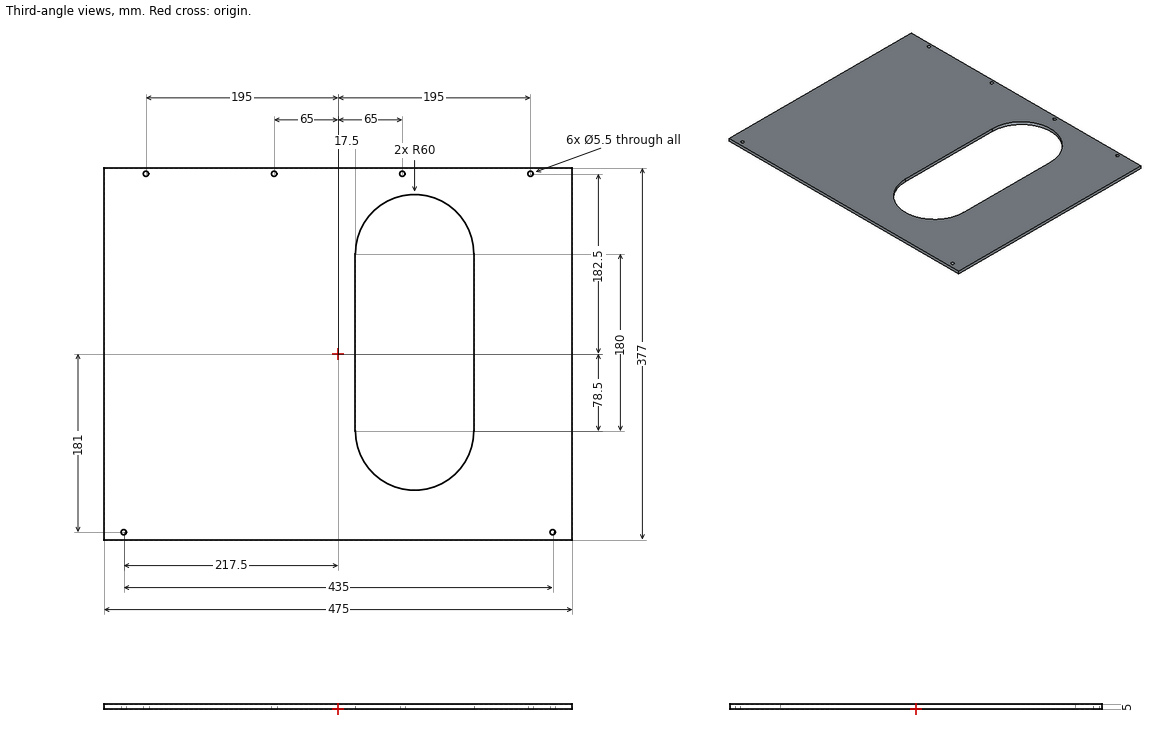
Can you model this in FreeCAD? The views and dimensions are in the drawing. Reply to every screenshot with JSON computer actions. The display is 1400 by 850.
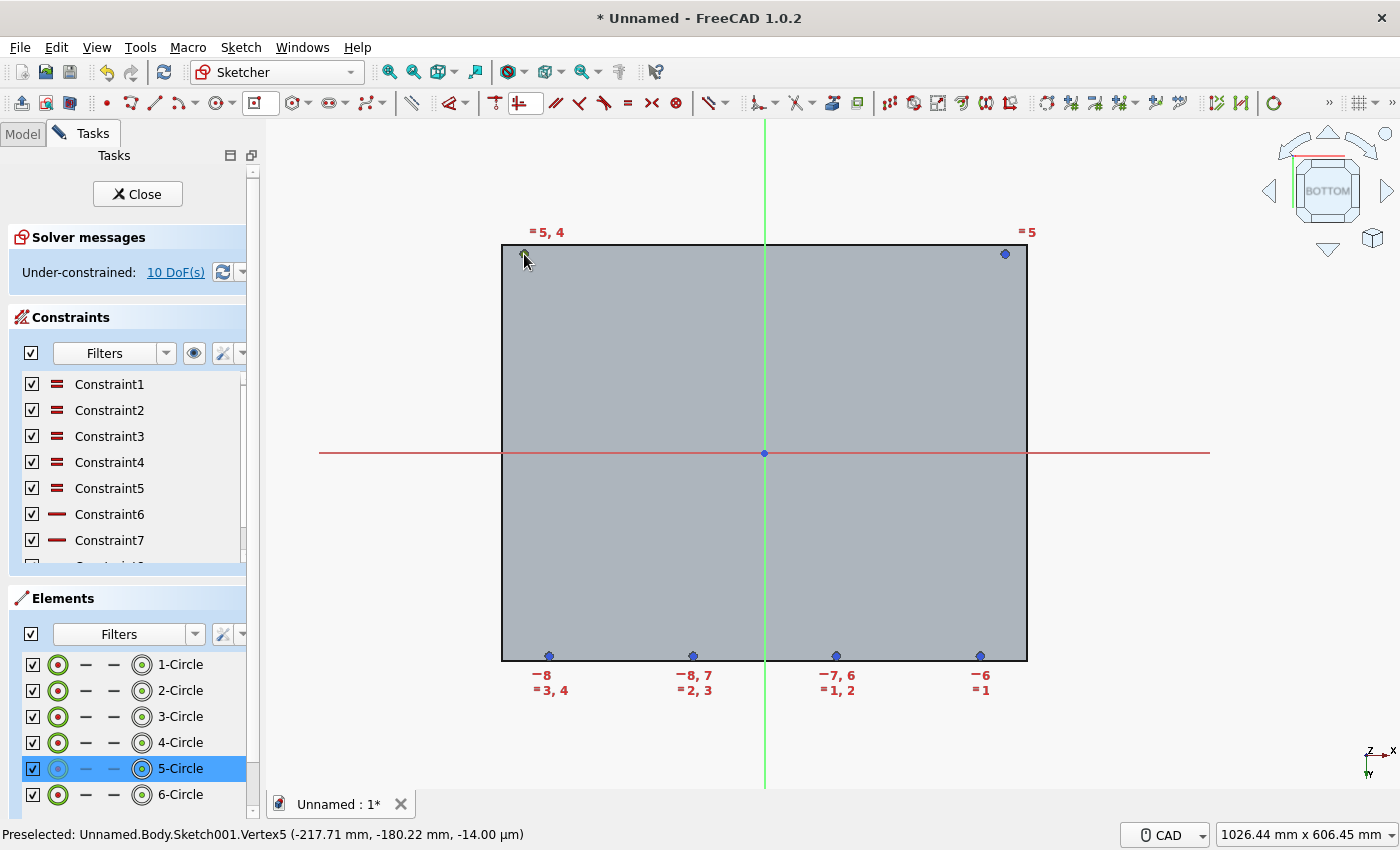
{"action": "left_click", "coordinate": [1005, 254]}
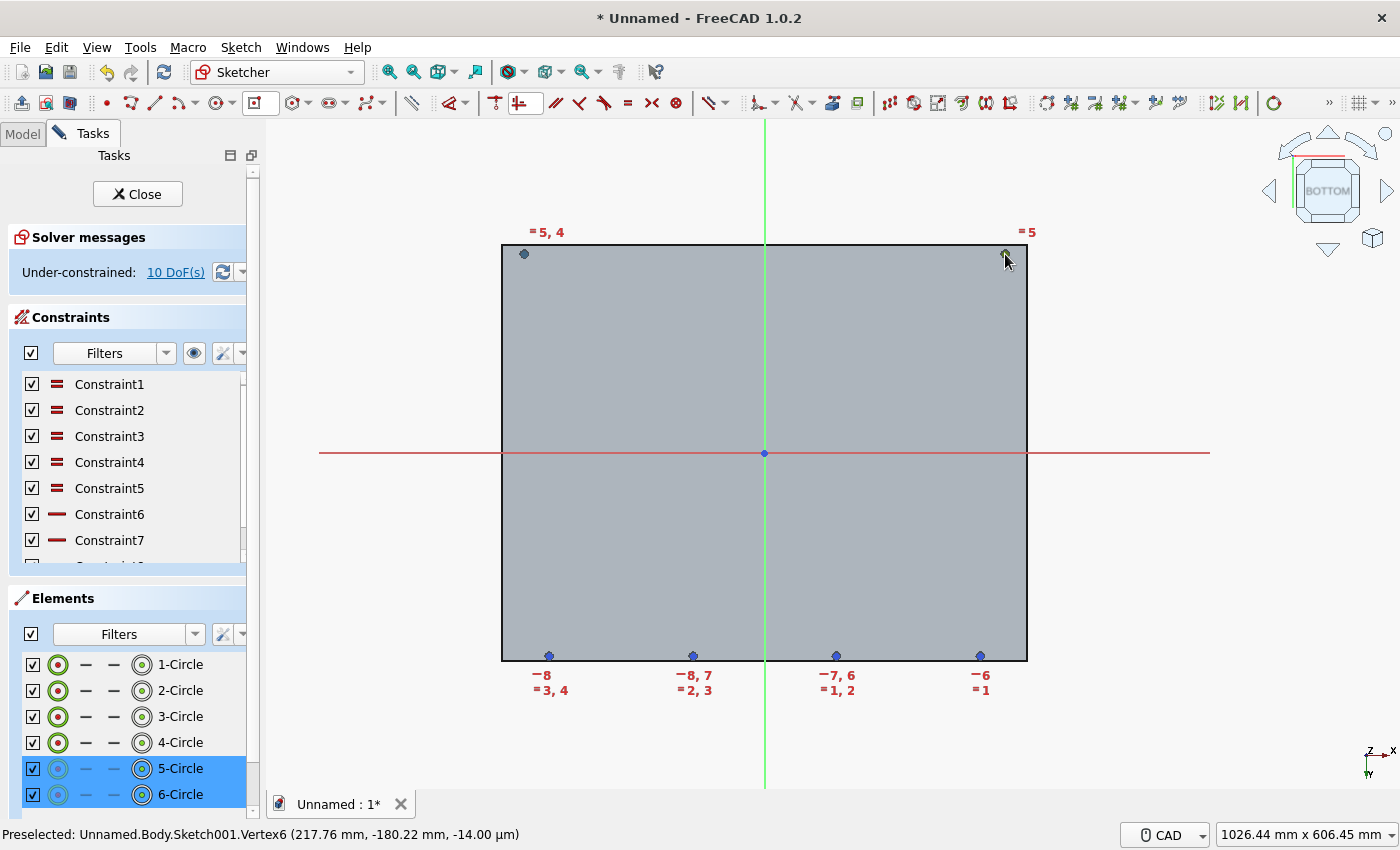
{"action": "key", "text": "h"}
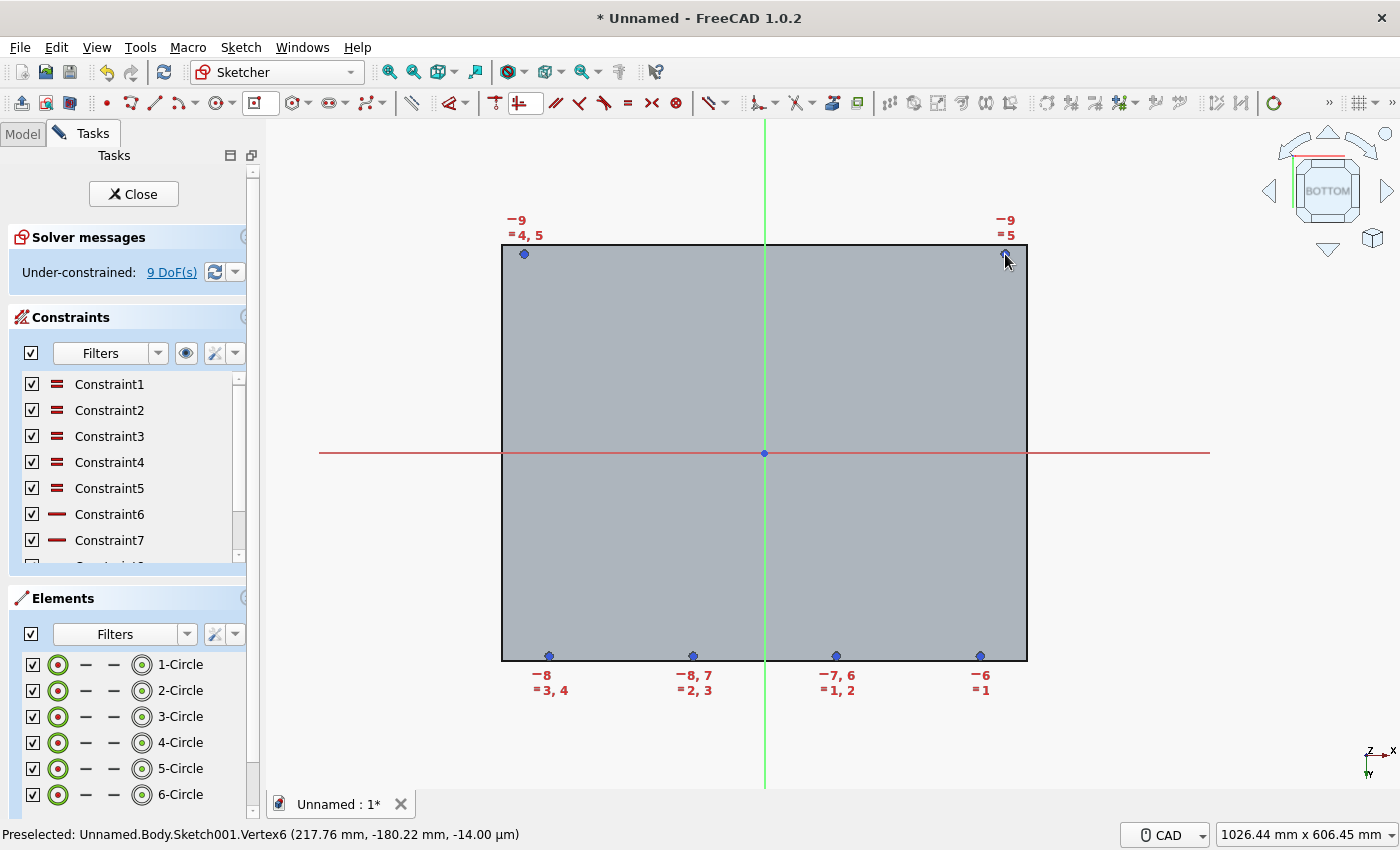
{"action": "scroll", "coordinate": [983, 653], "scroll_direction": "up", "scroll_amount": 10}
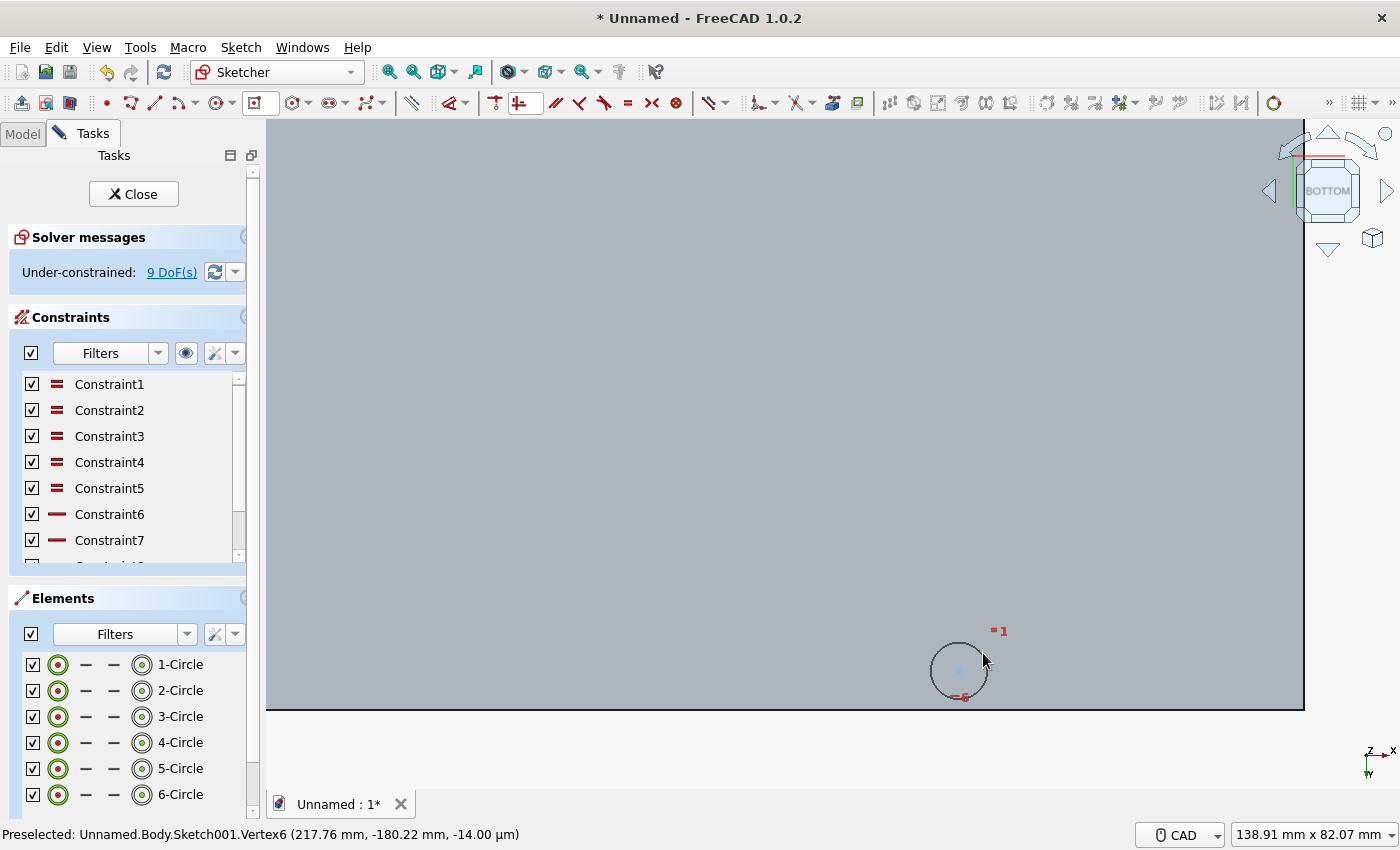
{"action": "left_click", "coordinate": [979, 651]}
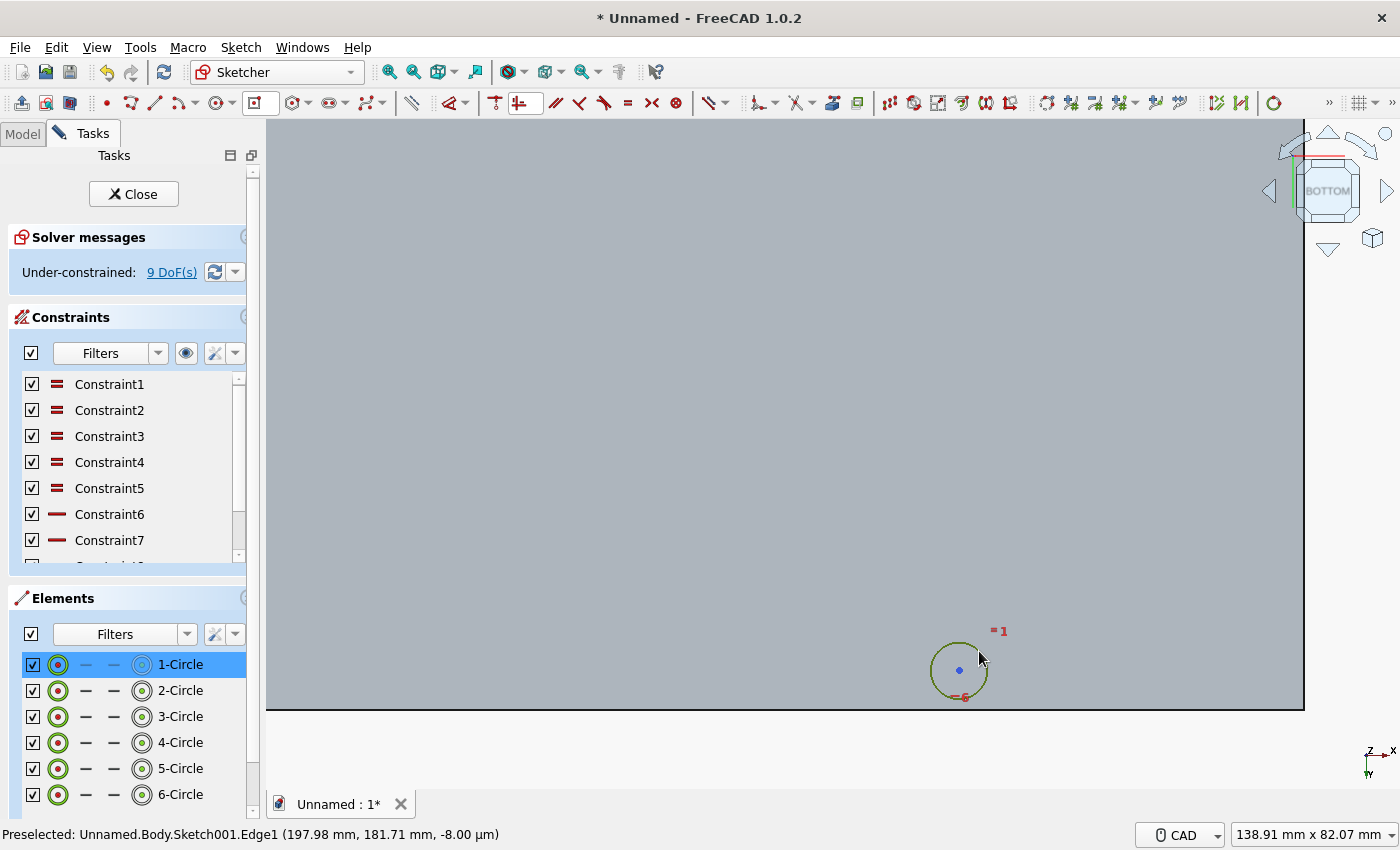
{"action": "key", "text": "k o"}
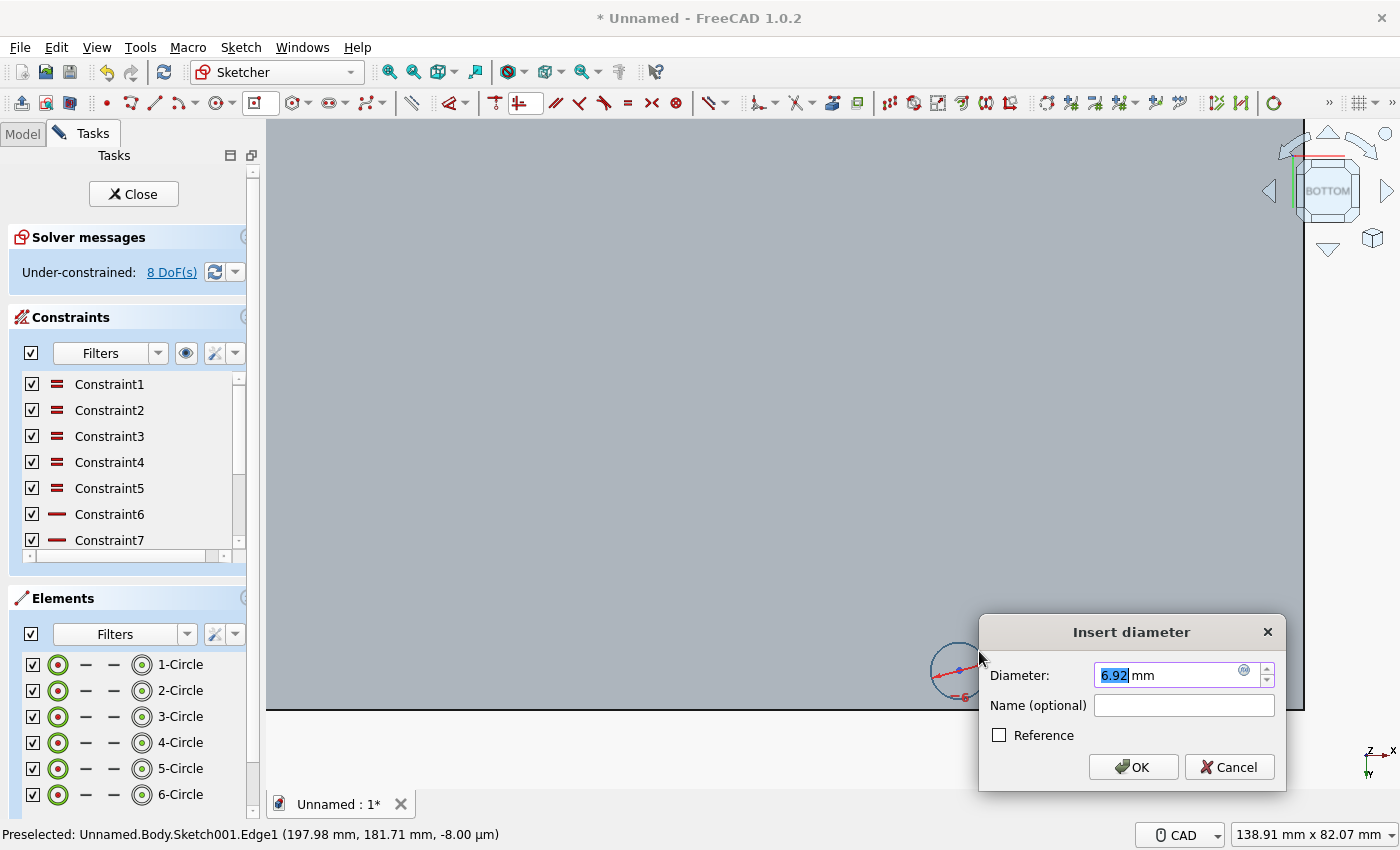
{"action": "type", "text": "5.5"}
{"action": "key", "text": "Return"}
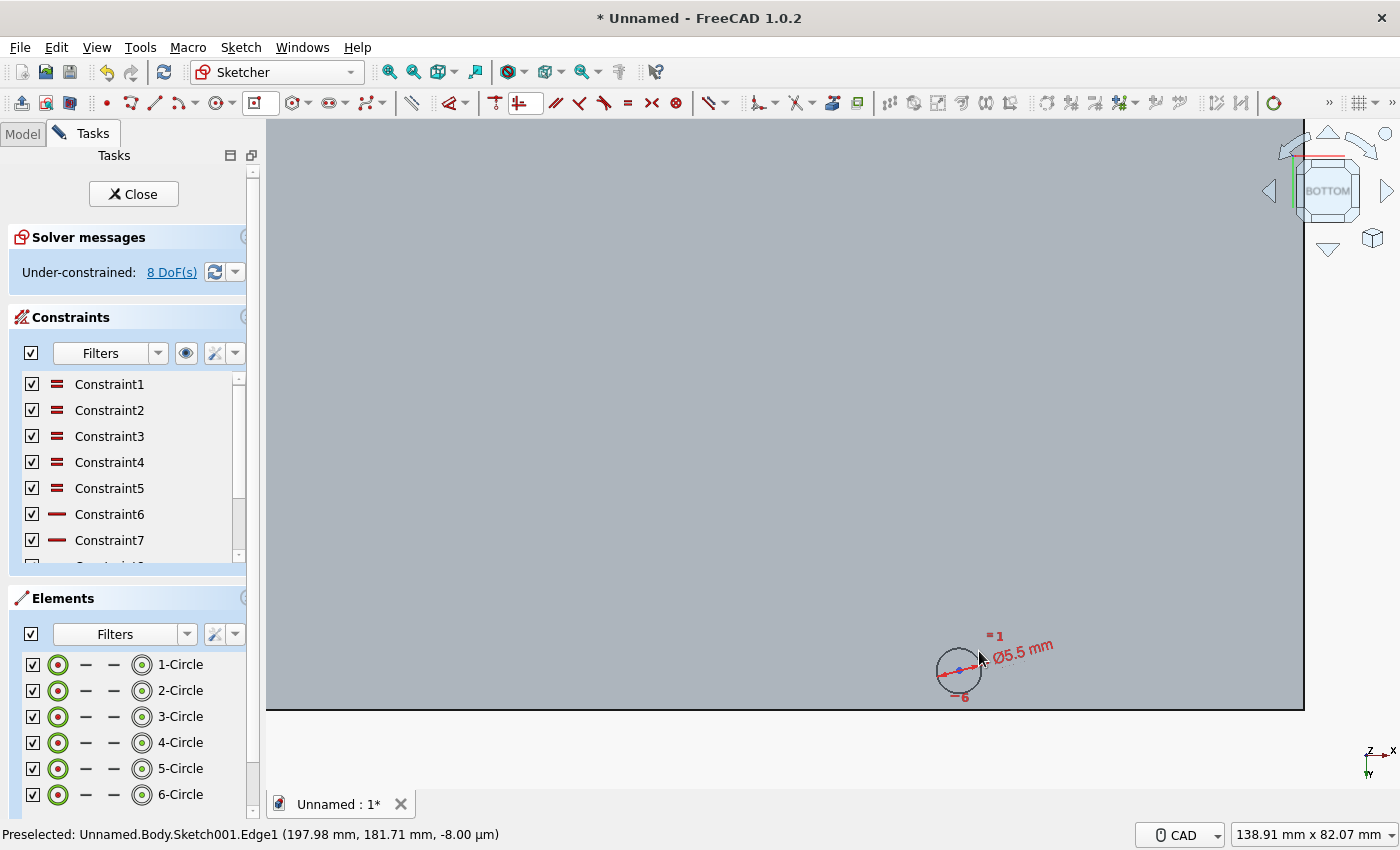
{"action": "scroll", "coordinate": [983, 654], "scroll_direction": "down", "scroll_amount": 10}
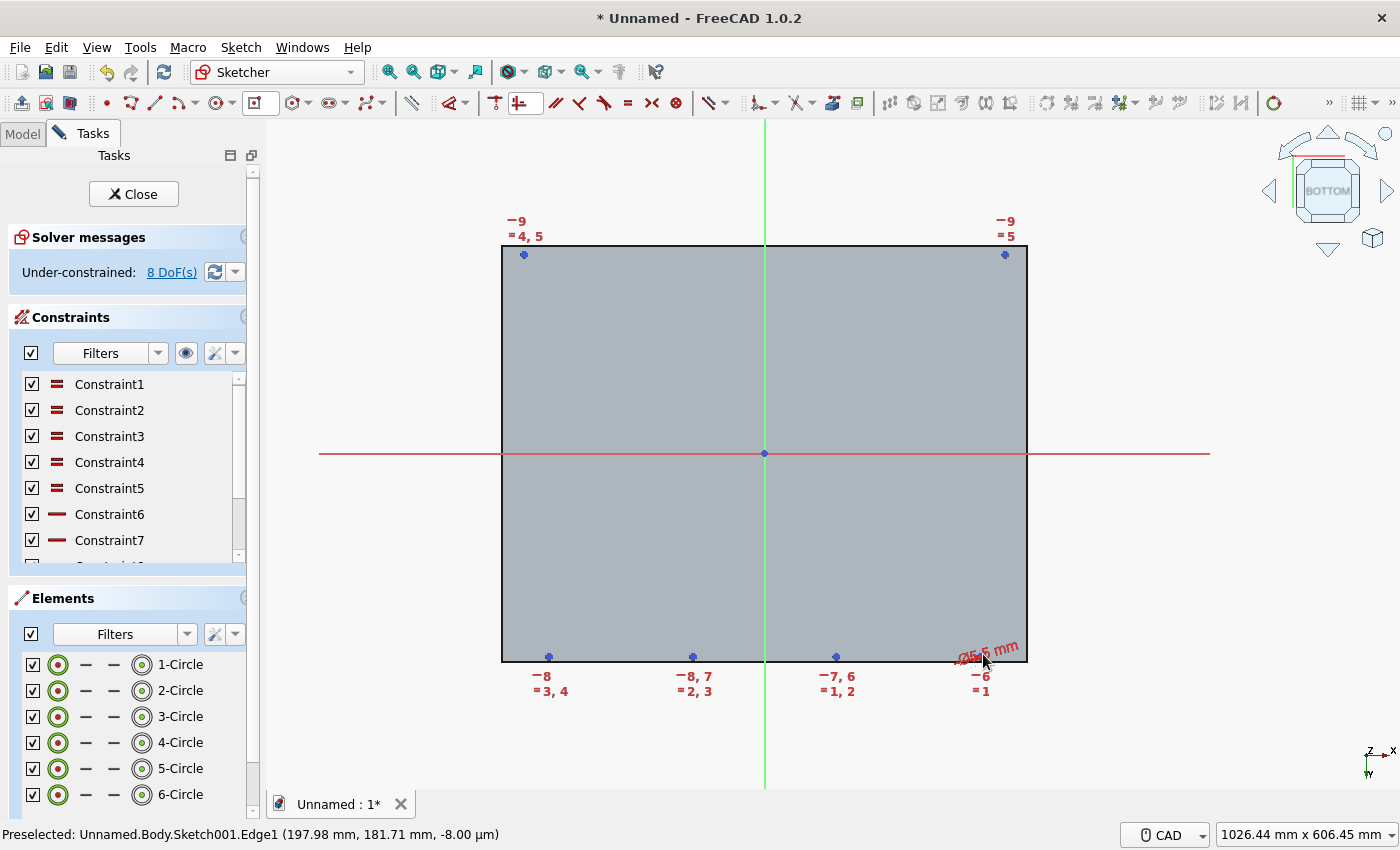
{"action": "left_click", "coordinate": [836, 657]}